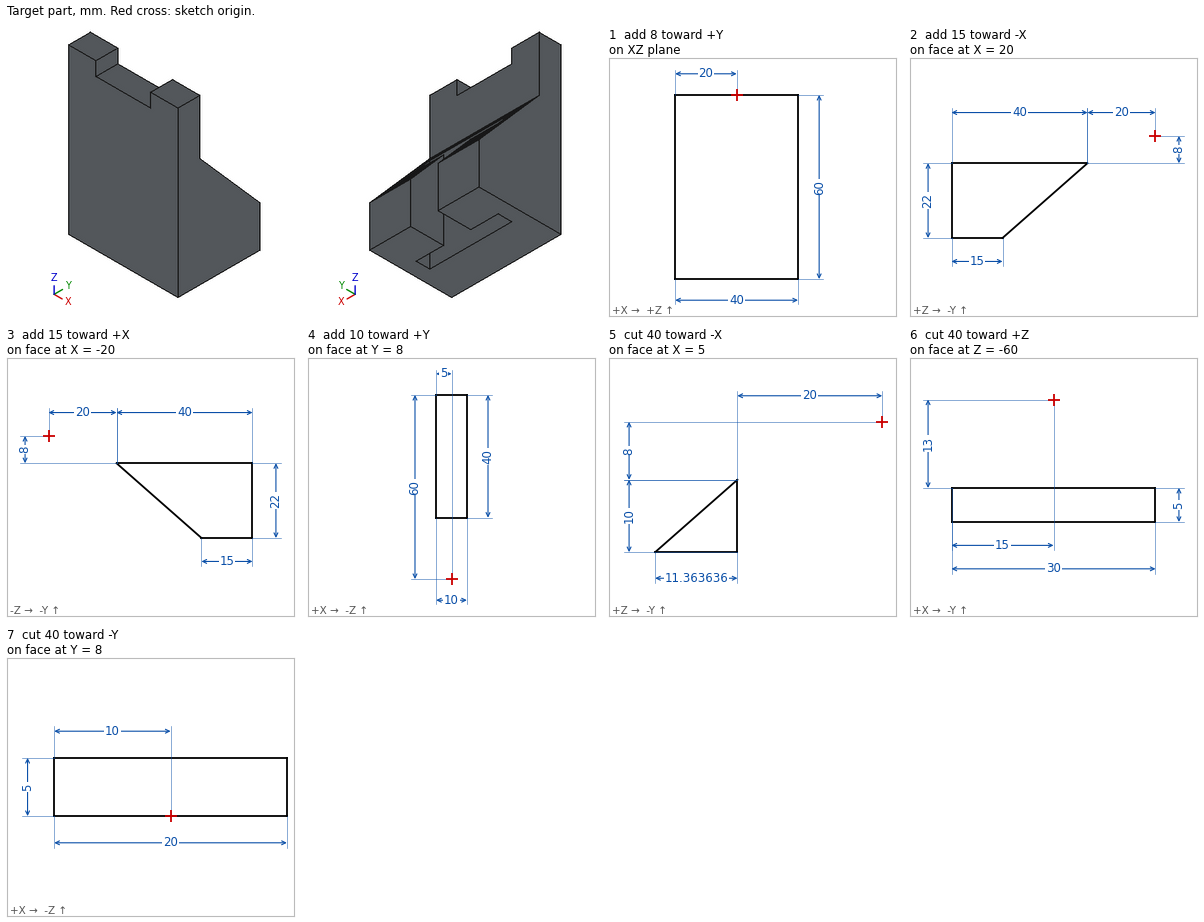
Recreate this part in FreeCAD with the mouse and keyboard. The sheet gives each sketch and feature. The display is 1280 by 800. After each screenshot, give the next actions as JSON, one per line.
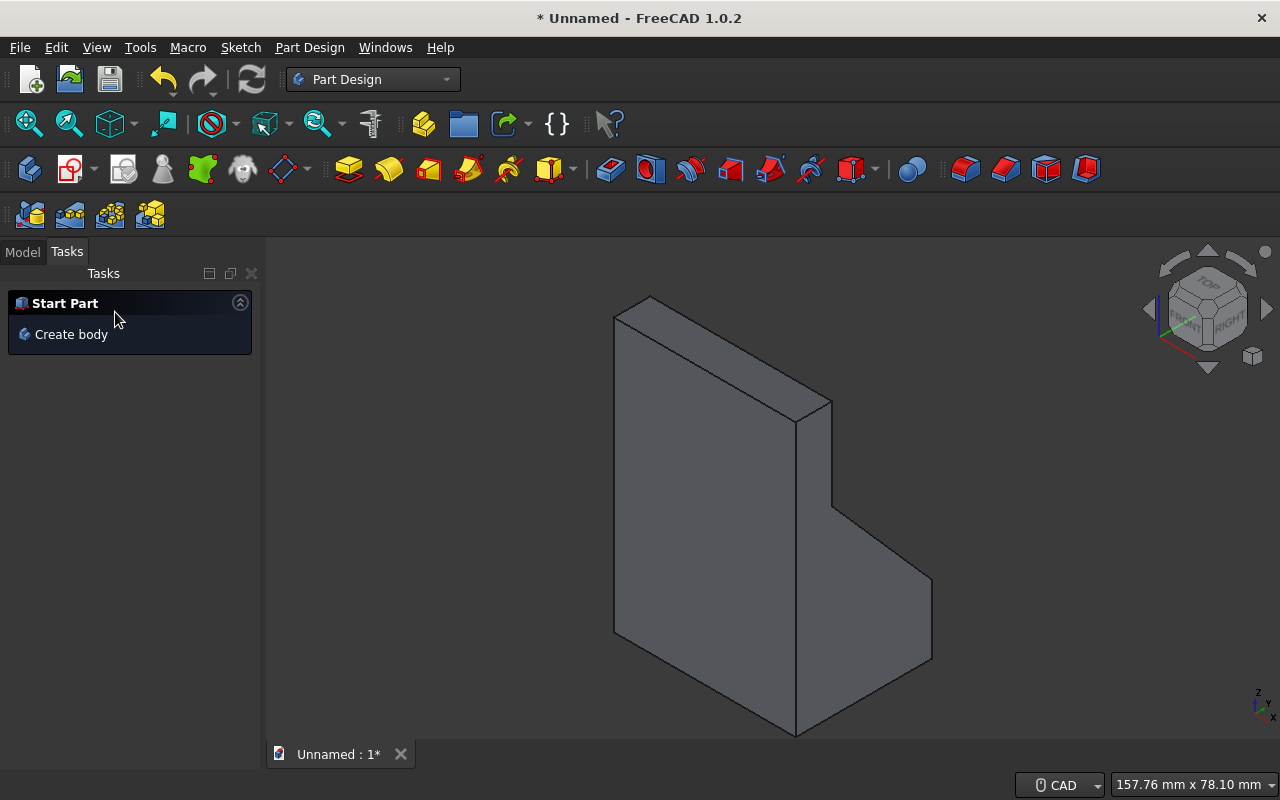
{"action": "key", "text": "3"}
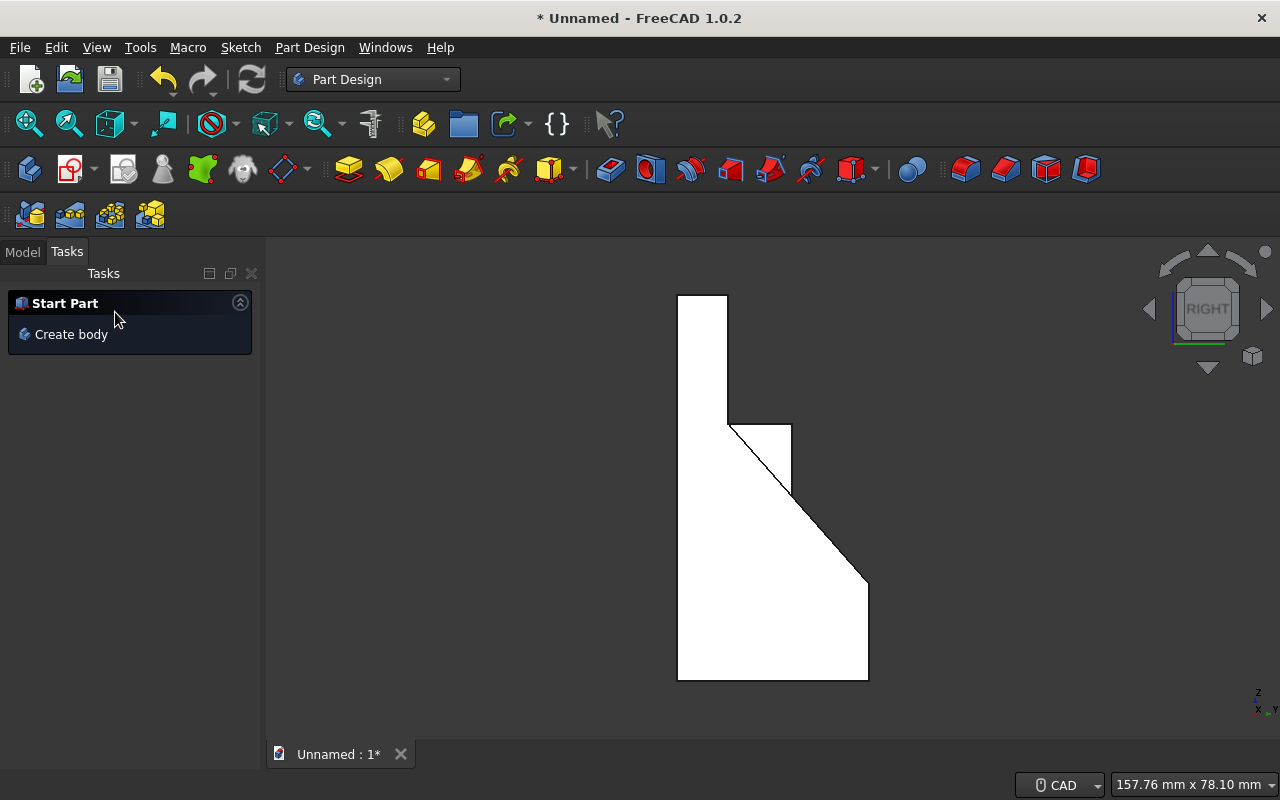
{"action": "left_click", "coordinate": [769, 438]}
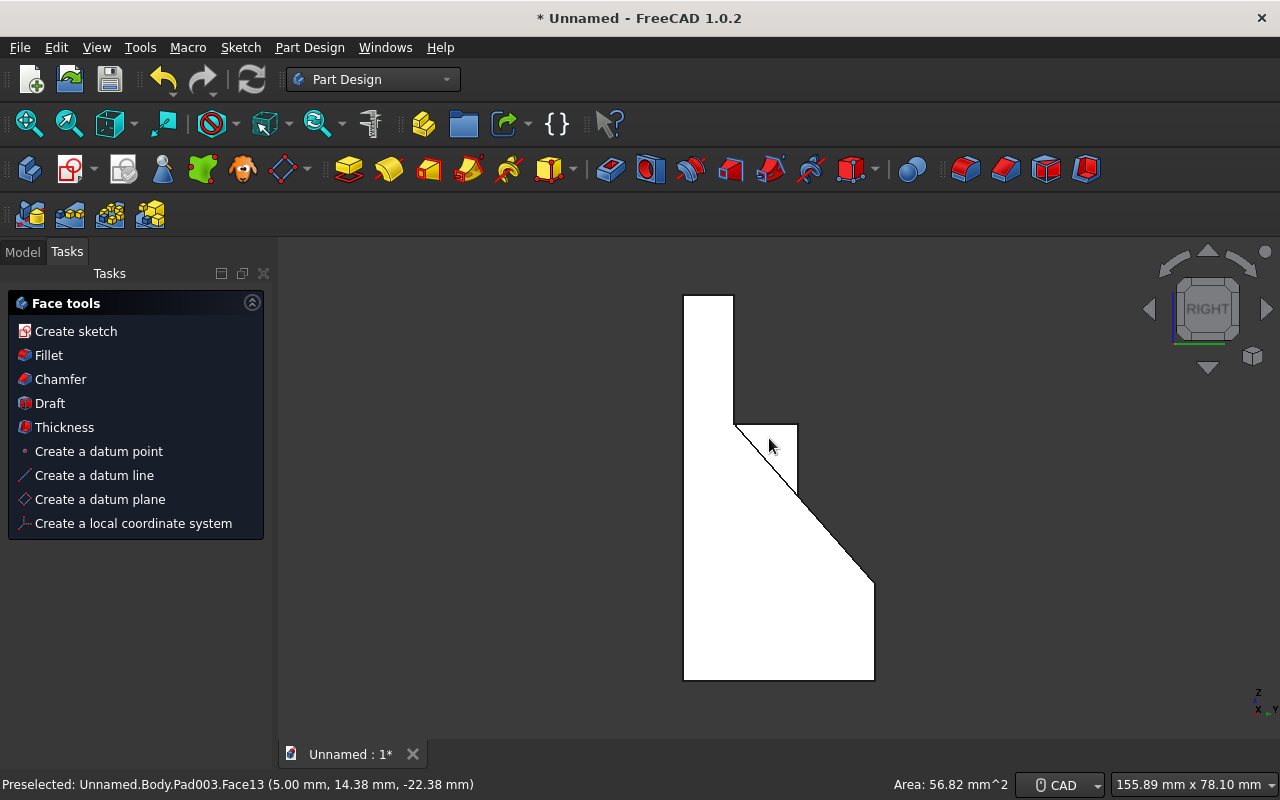
{"action": "left_click", "coordinate": [70, 170]}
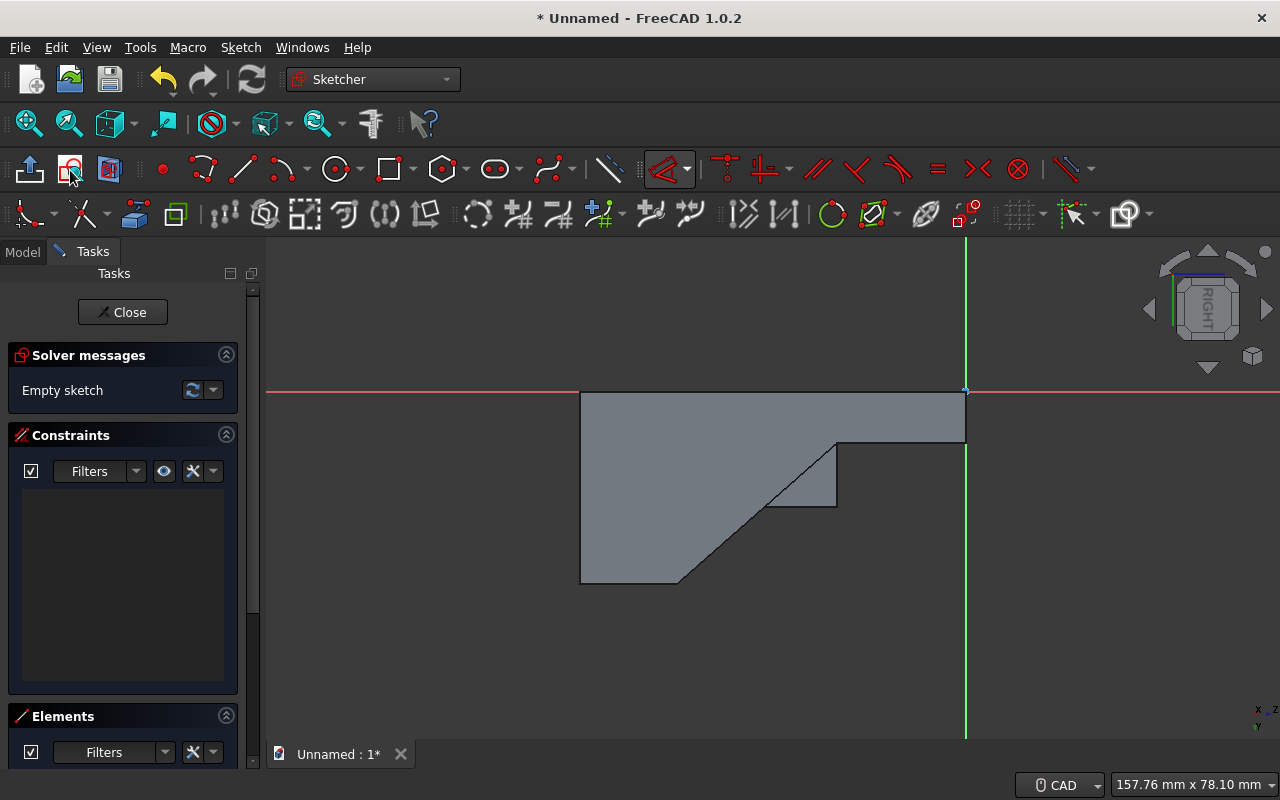
{"action": "left_click", "coordinate": [110, 170]}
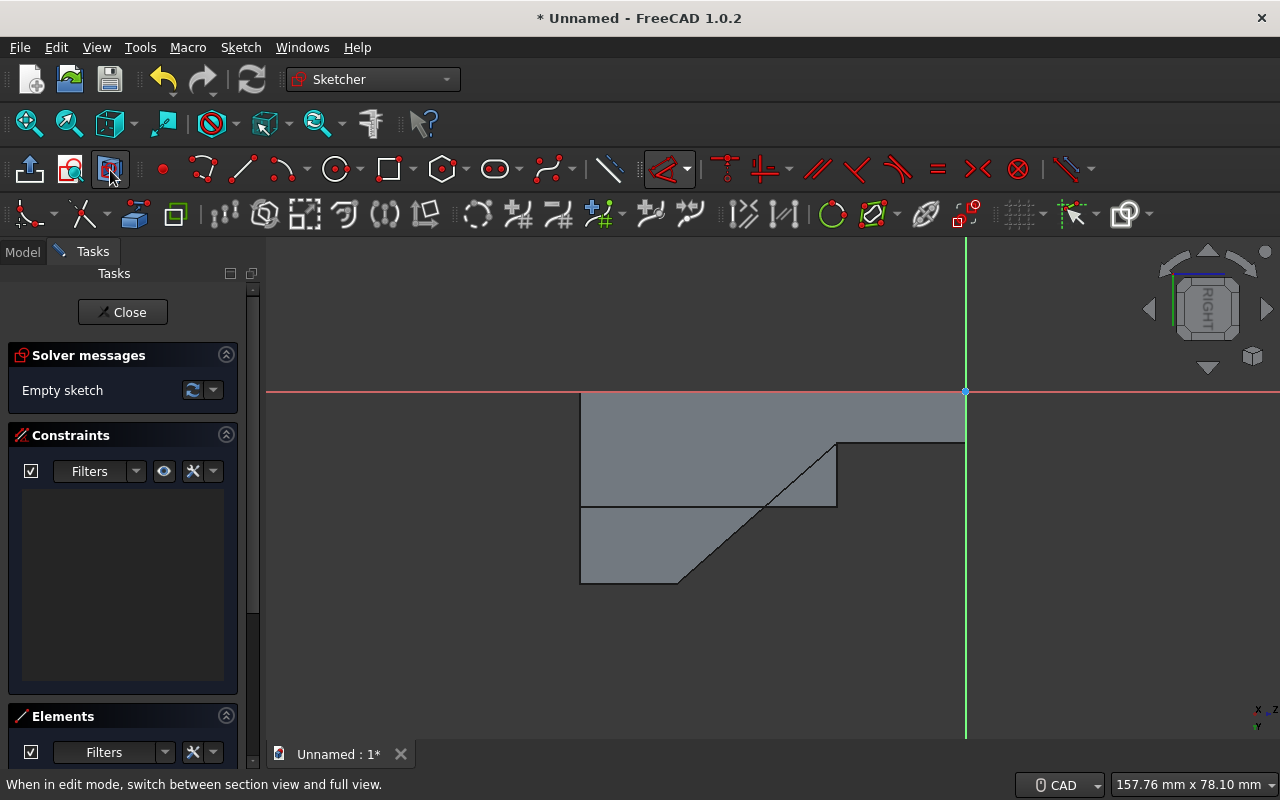
{"action": "scroll", "coordinate": [825, 472], "scroll_direction": "up", "scroll_amount": 8}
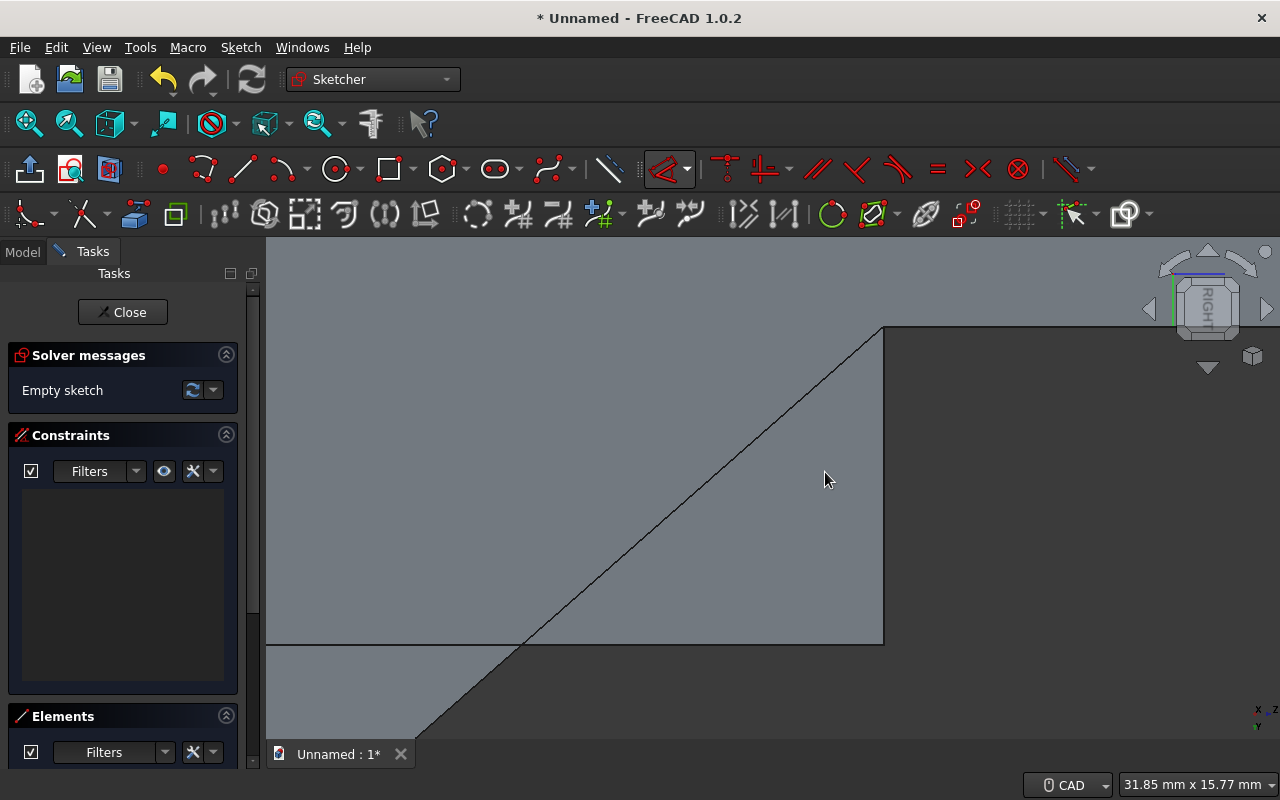
{"action": "left_click", "coordinate": [204, 170]}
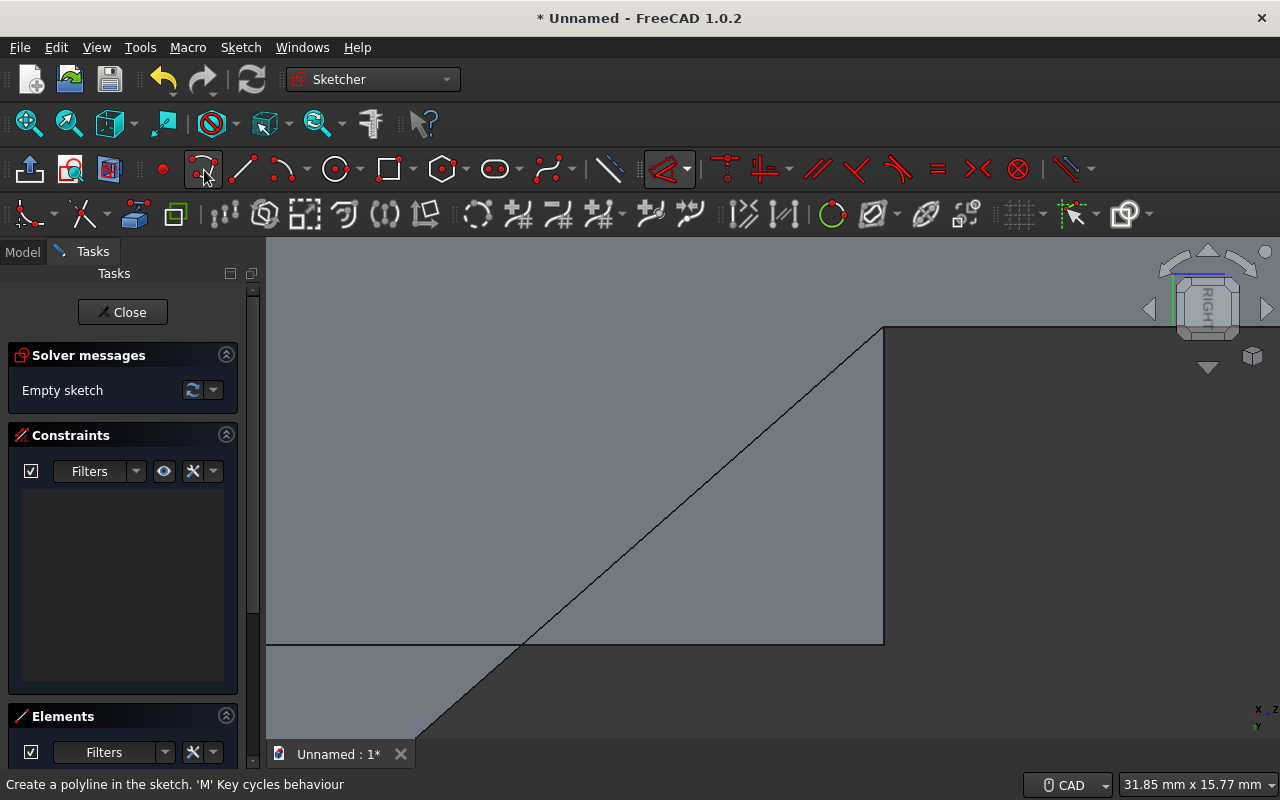
{"action": "left_click", "coordinate": [884, 327]}
{"action": "left_click", "coordinate": [522, 645]}
{"action": "left_click", "coordinate": [884, 645]}
{"action": "left_click", "coordinate": [884, 328]}
{"action": "key", "text": "Escape"}
{"action": "key", "text": "Escape"}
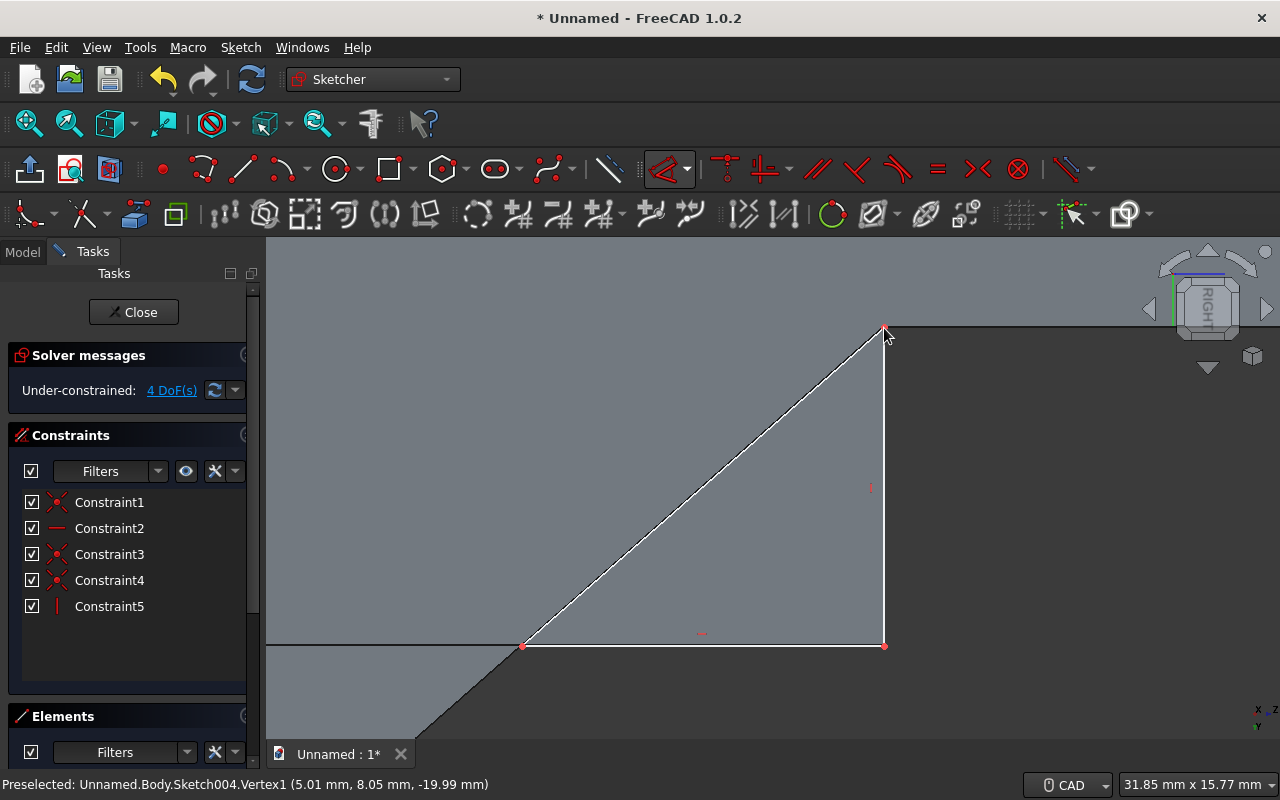
{"action": "left_click", "coordinate": [884, 551]}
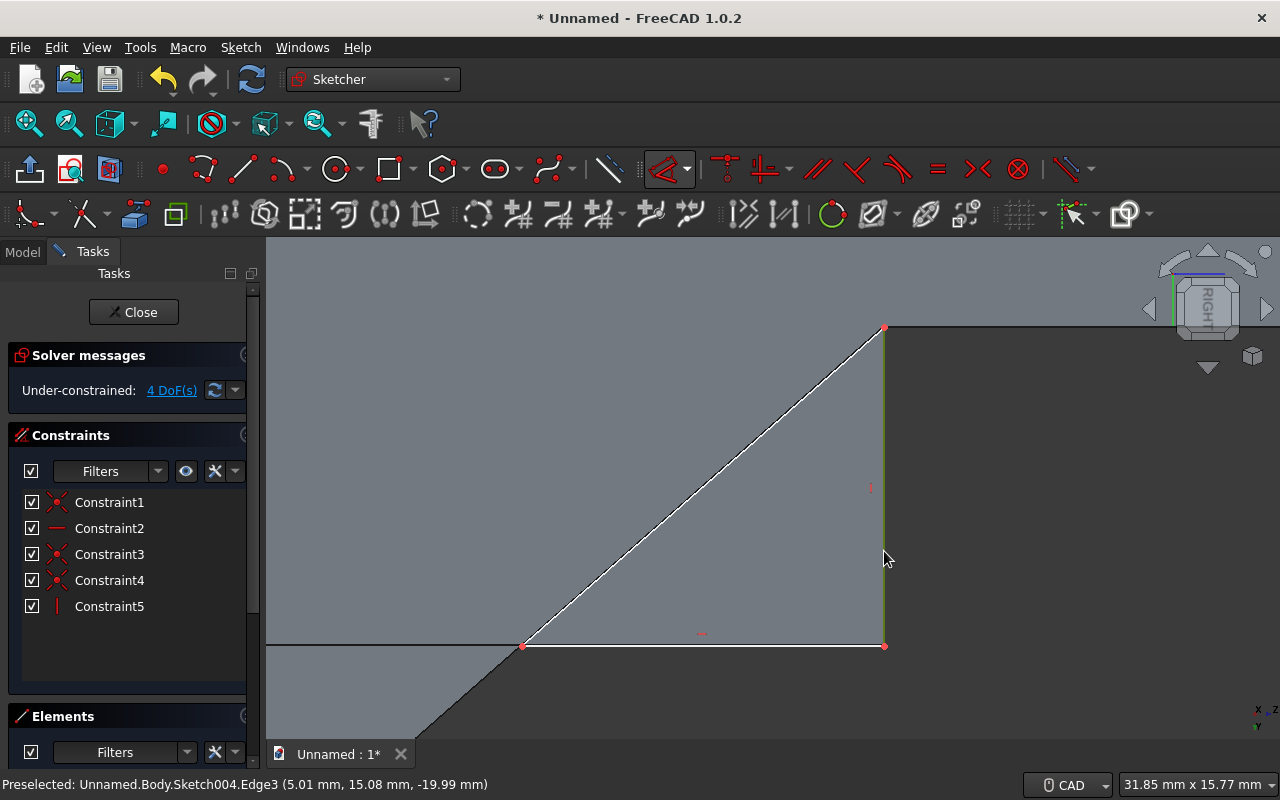
{"action": "left_click", "coordinate": [690, 170]}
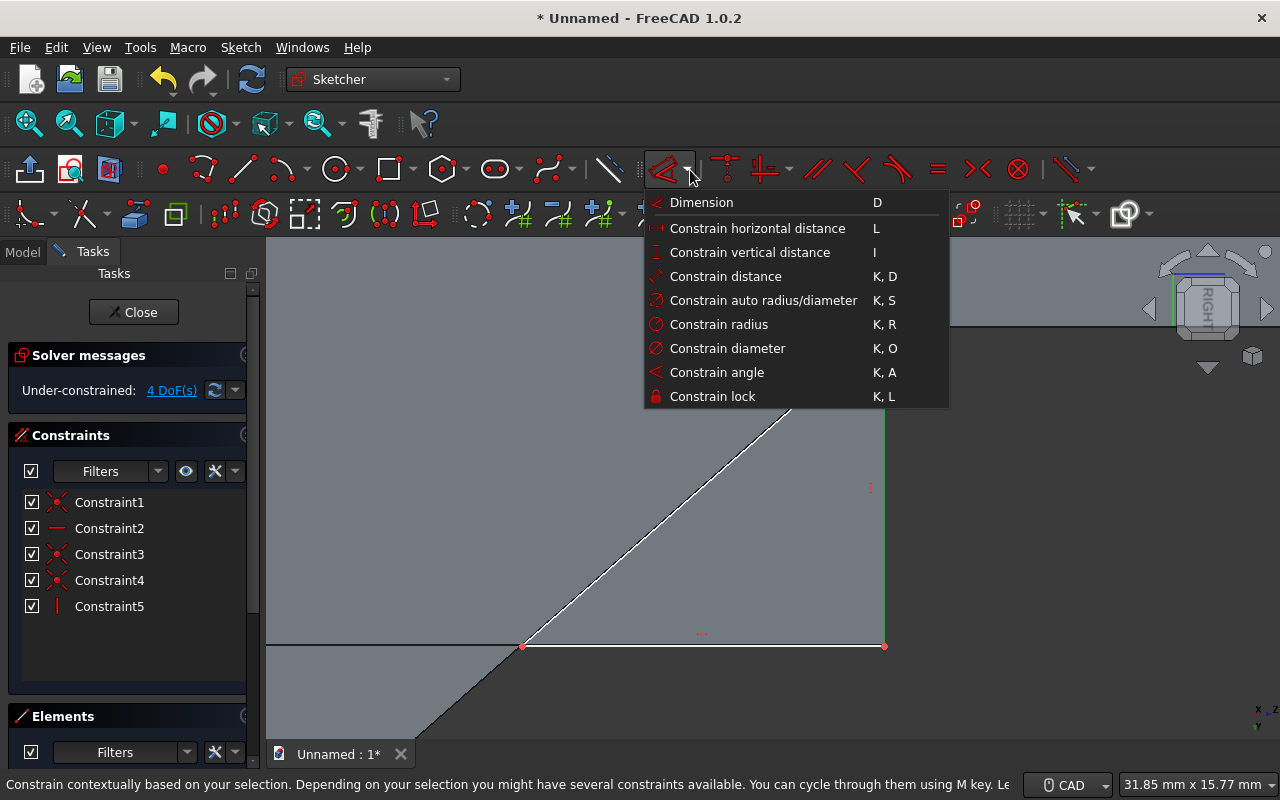
{"action": "left_click", "coordinate": [797, 252]}